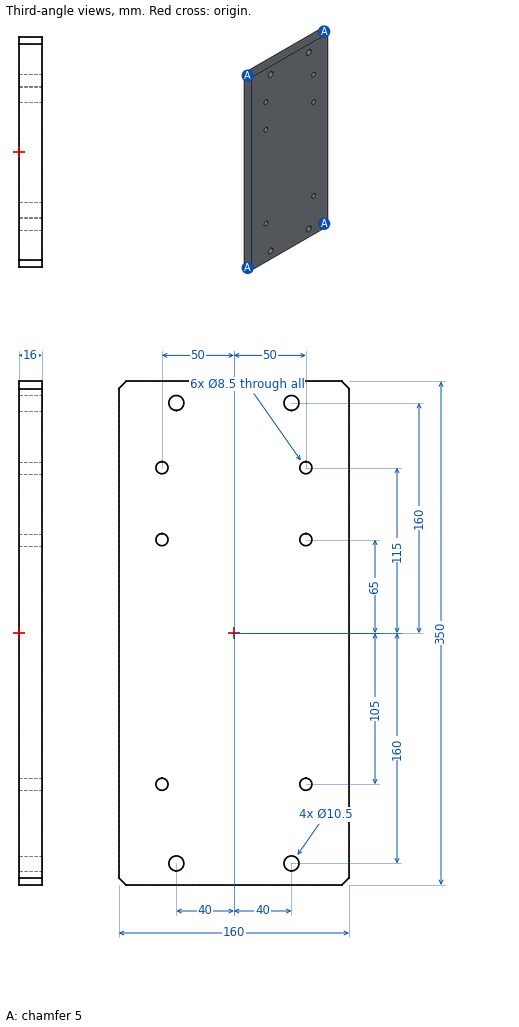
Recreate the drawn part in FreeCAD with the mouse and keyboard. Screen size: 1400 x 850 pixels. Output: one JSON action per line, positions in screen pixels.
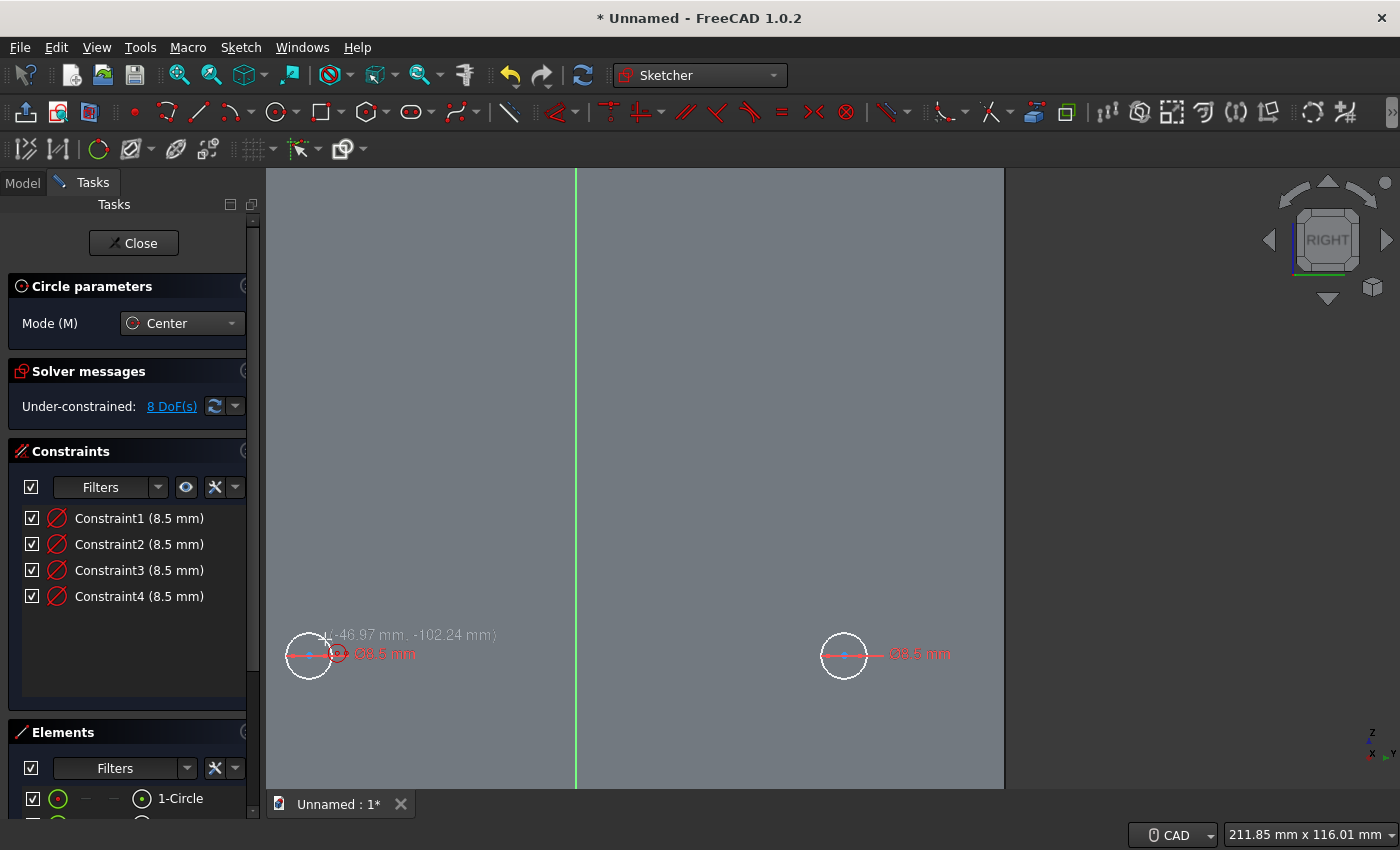
{"action": "scroll", "coordinate": [846, 656], "scroll_direction": "down", "scroll_amount": 6}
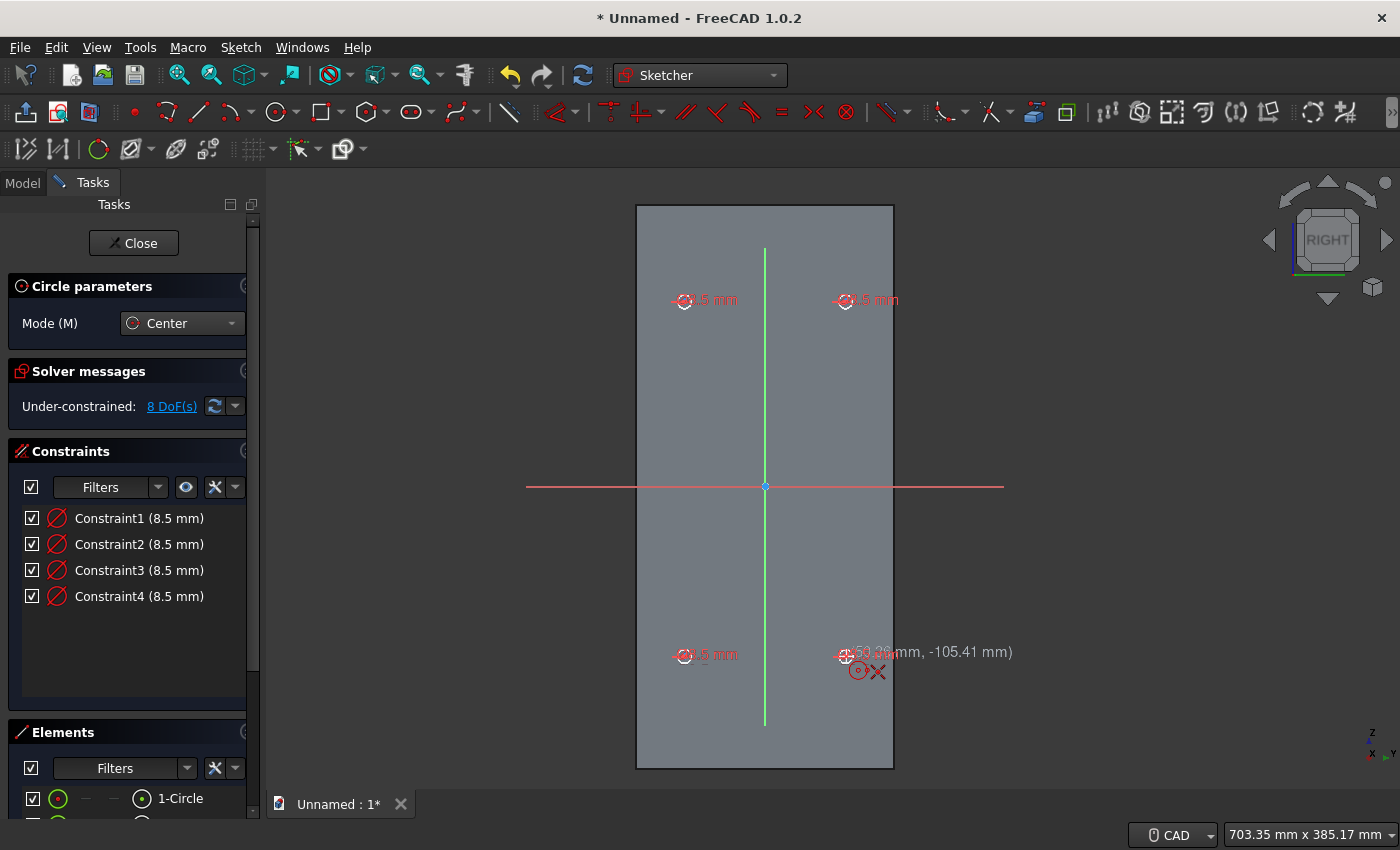
{"action": "scroll", "coordinate": [846, 382], "scroll_direction": "up", "scroll_amount": 6}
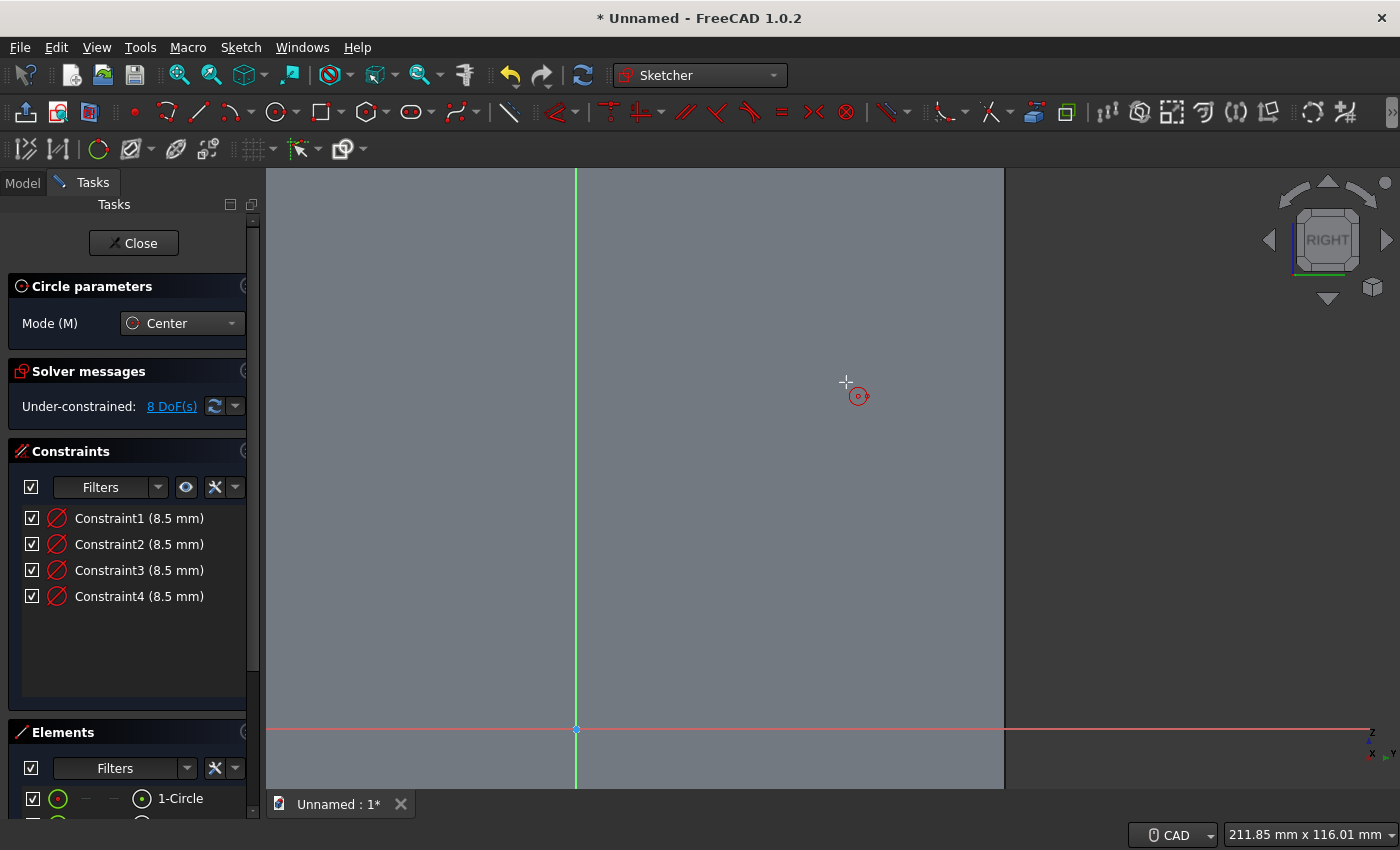
{"action": "left_click", "coordinate": [844, 382]}
{"action": "mouse_move", "coordinate": [860, 365]}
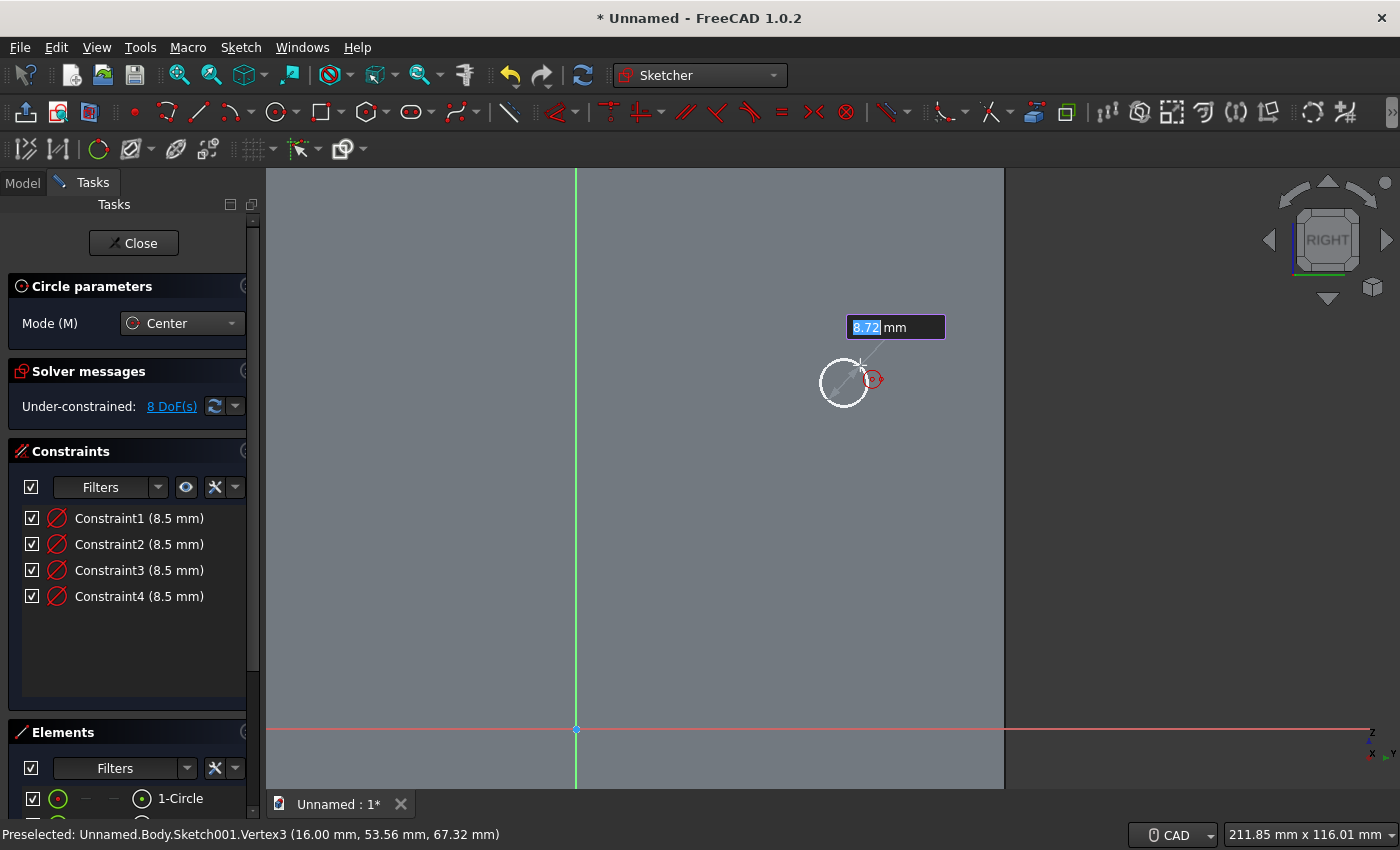
{"action": "type", "text": "8.5"}
{"action": "key", "text": "Return"}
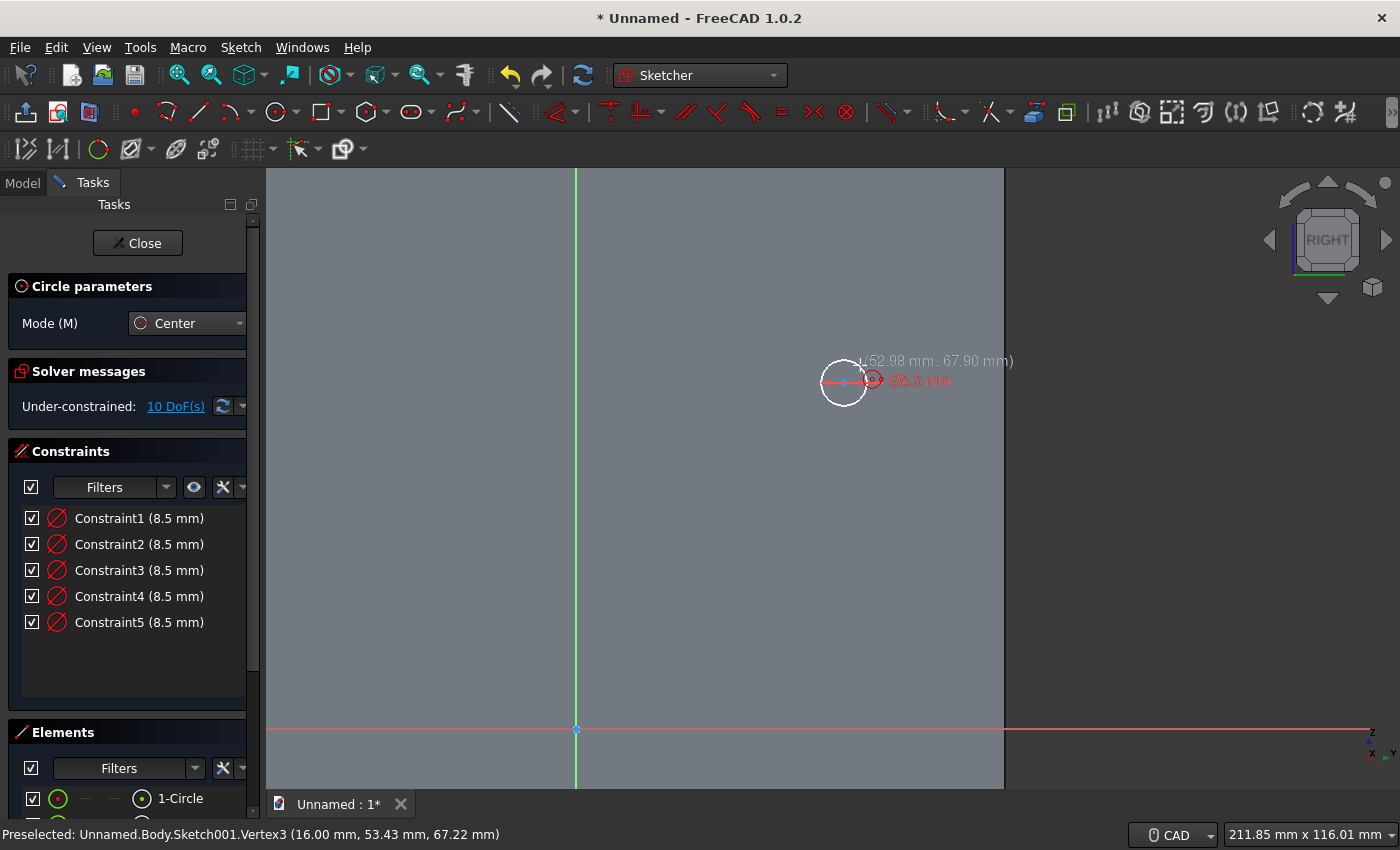
{"action": "left_click", "coordinate": [309, 382]}
{"action": "mouse_move", "coordinate": [325, 365]}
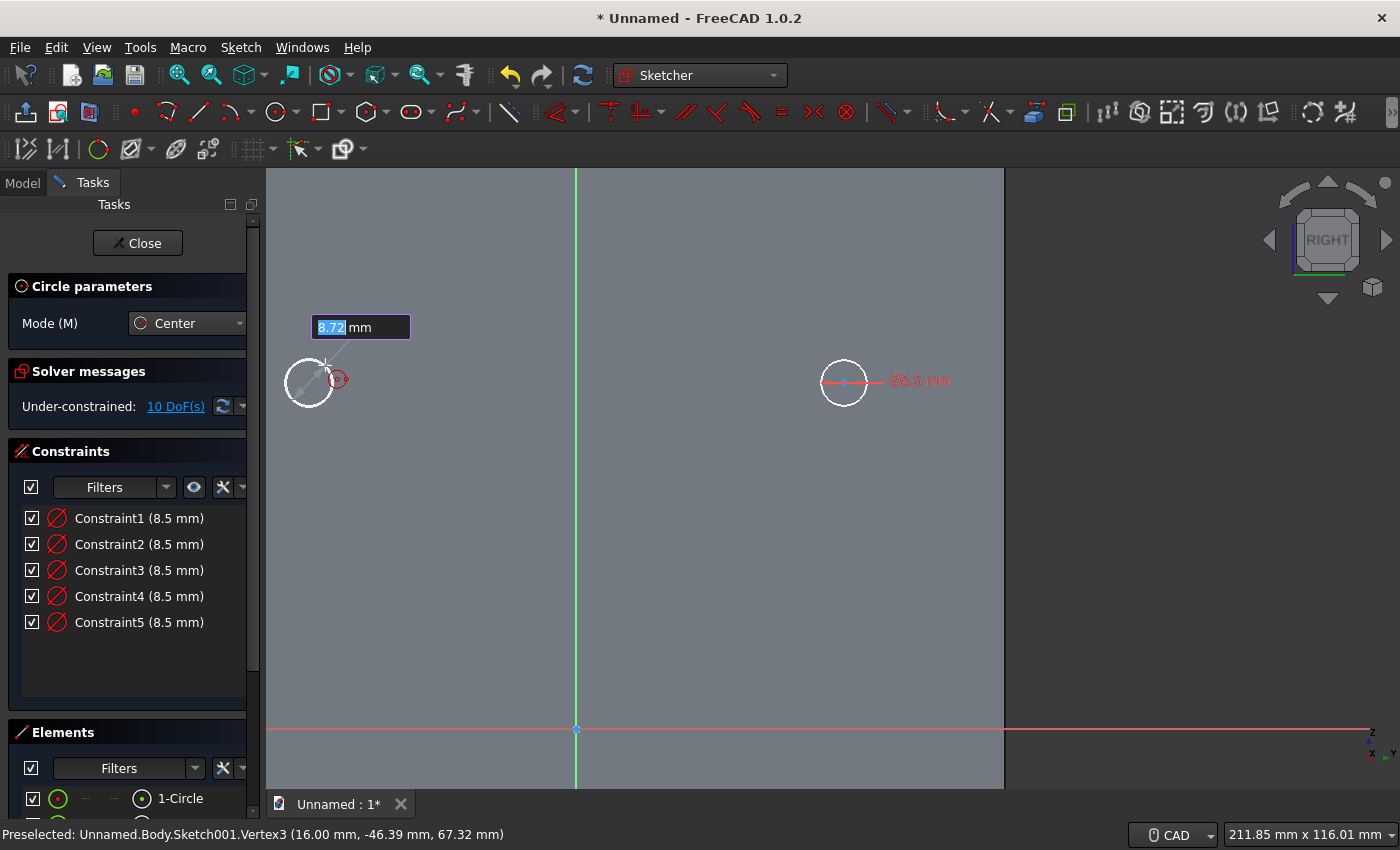
{"action": "type", "text": "8.5"}
{"action": "key", "text": "Return"}
{"action": "key", "text": "Escape"}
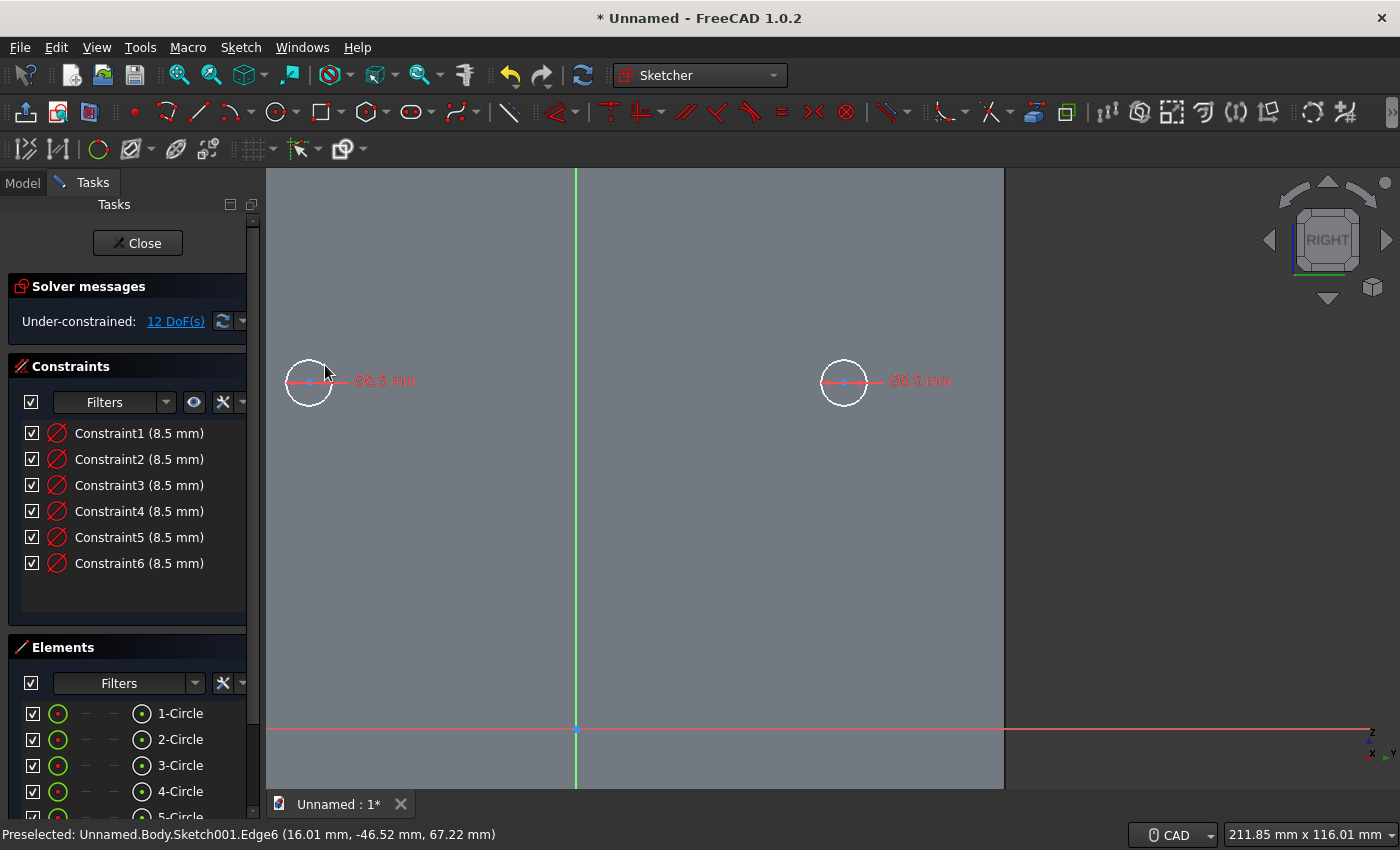
{"action": "scroll", "coordinate": [846, 382], "scroll_direction": "down", "scroll_amount": 6}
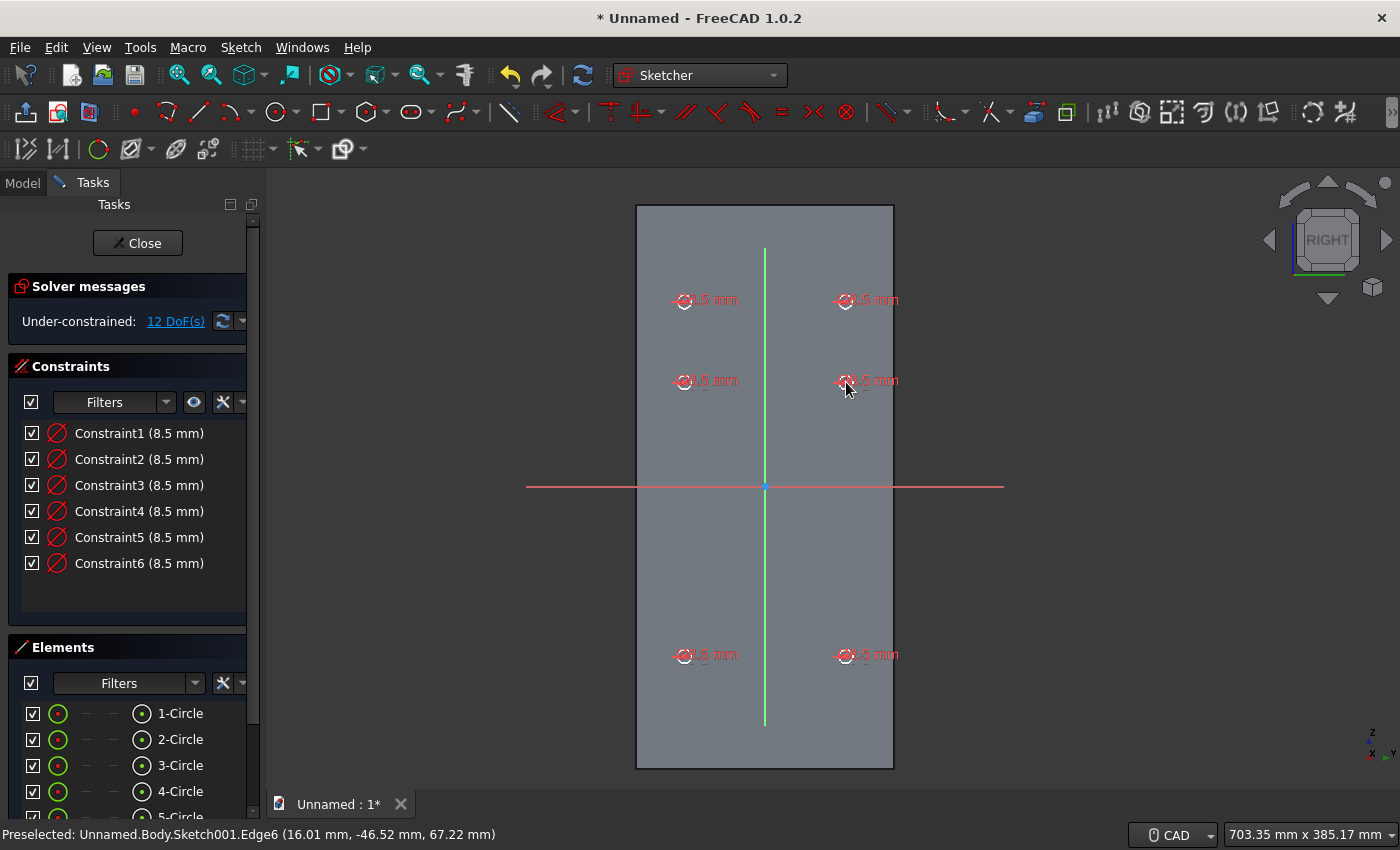
{"action": "left_click", "coordinate": [846, 302]}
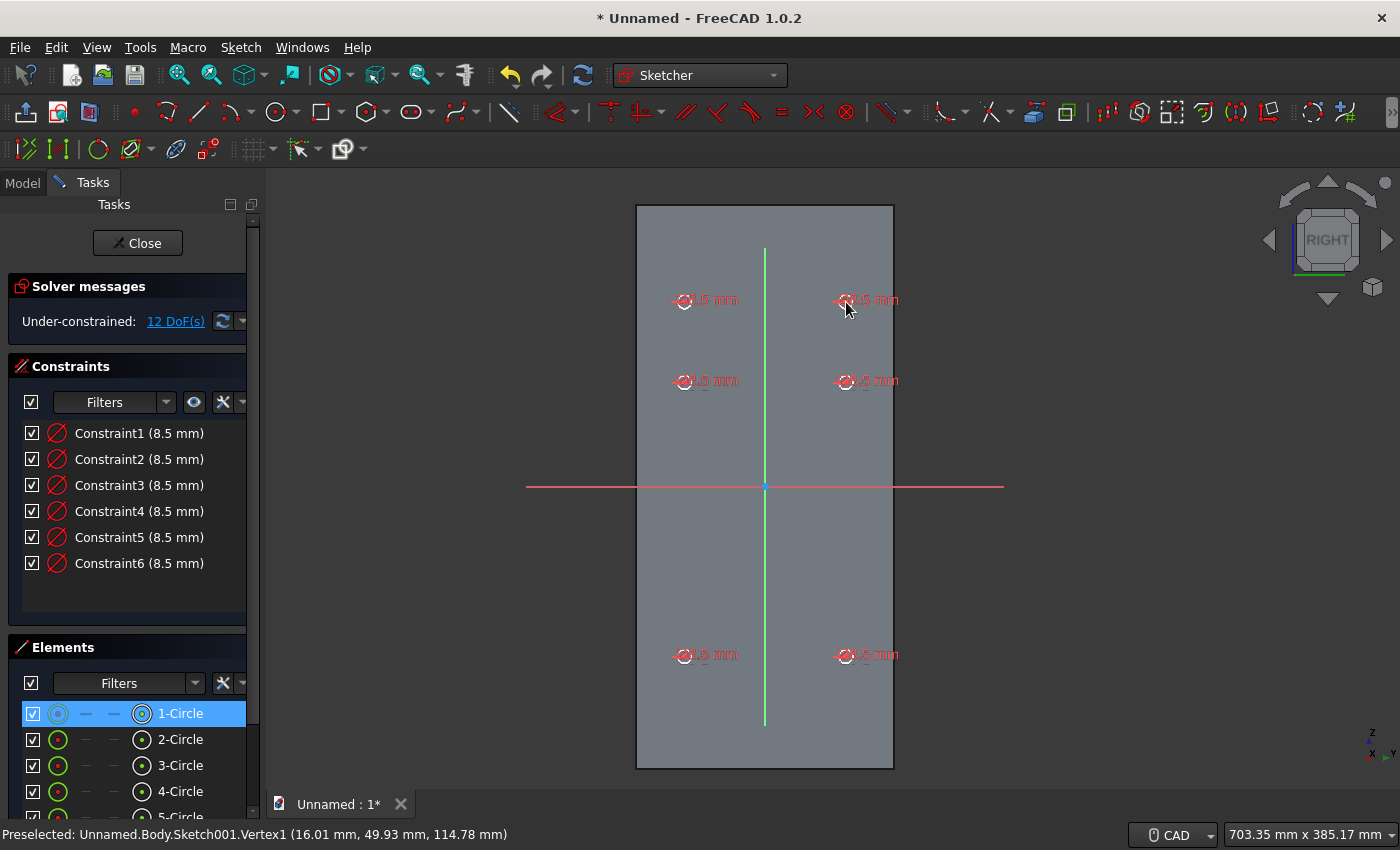
{"action": "left_click", "coordinate": [685, 302]}